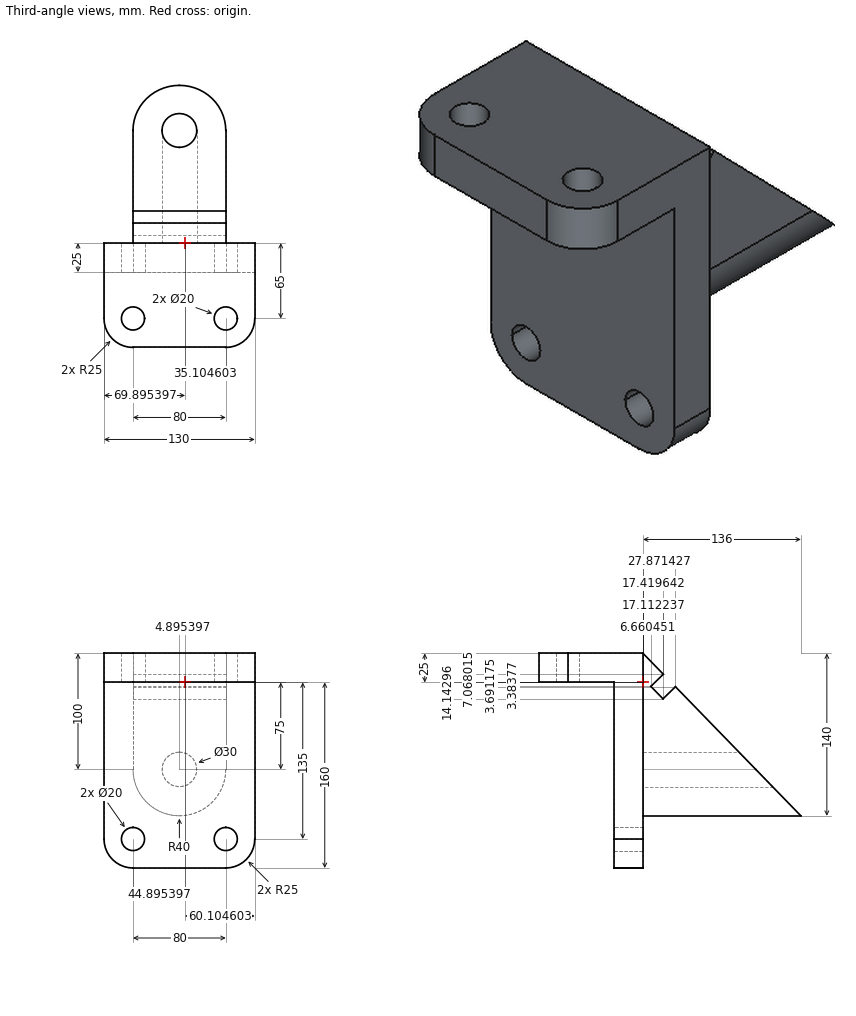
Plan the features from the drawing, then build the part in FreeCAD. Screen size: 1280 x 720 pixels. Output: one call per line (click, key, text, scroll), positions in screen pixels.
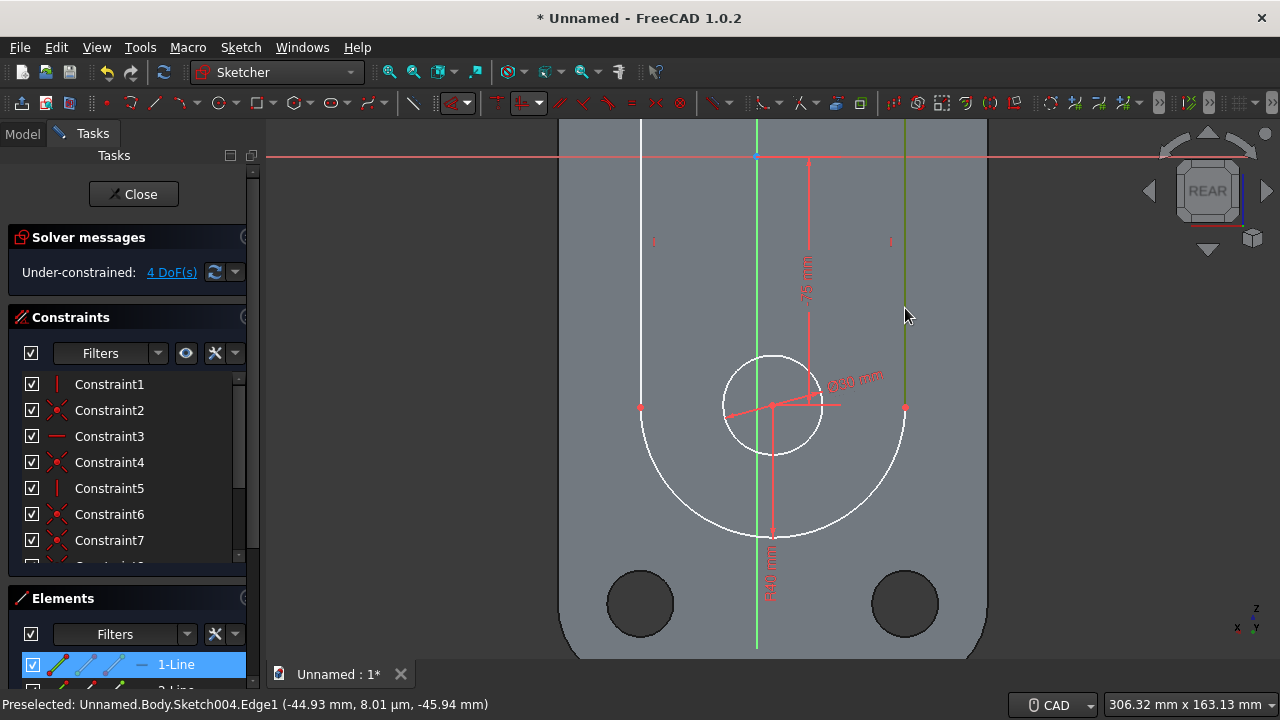
click(470, 104)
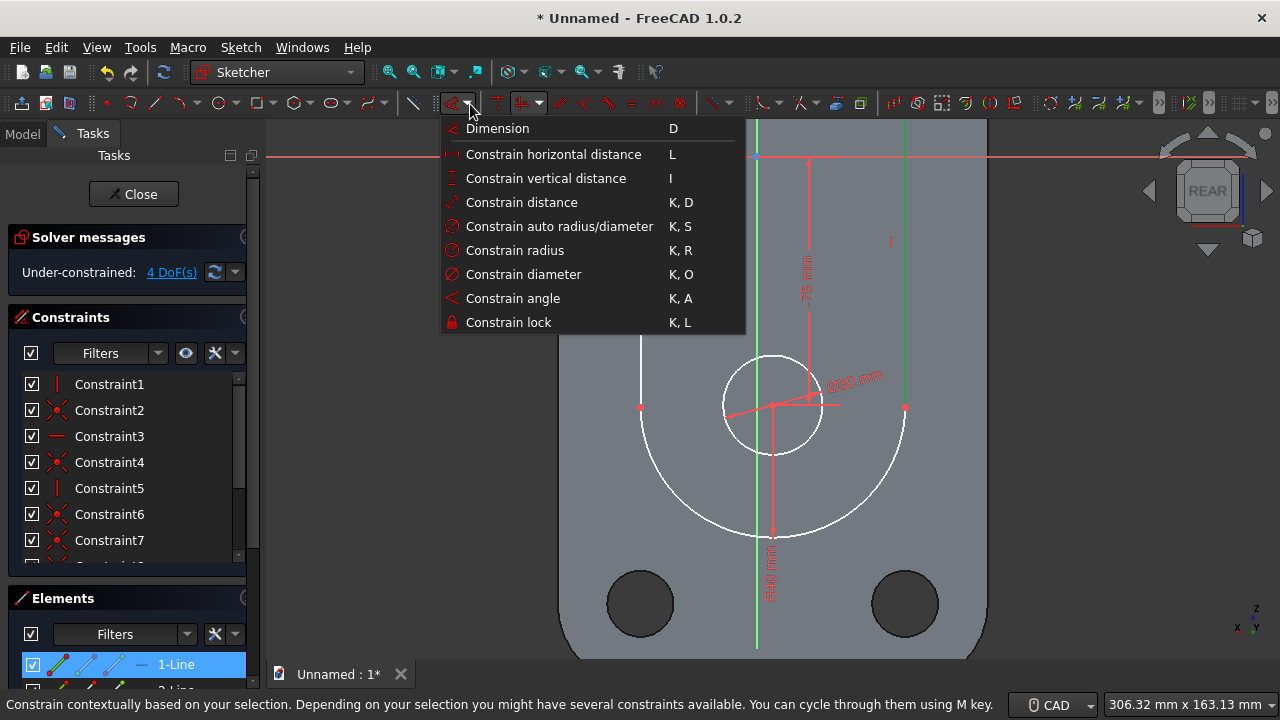
click(593, 178)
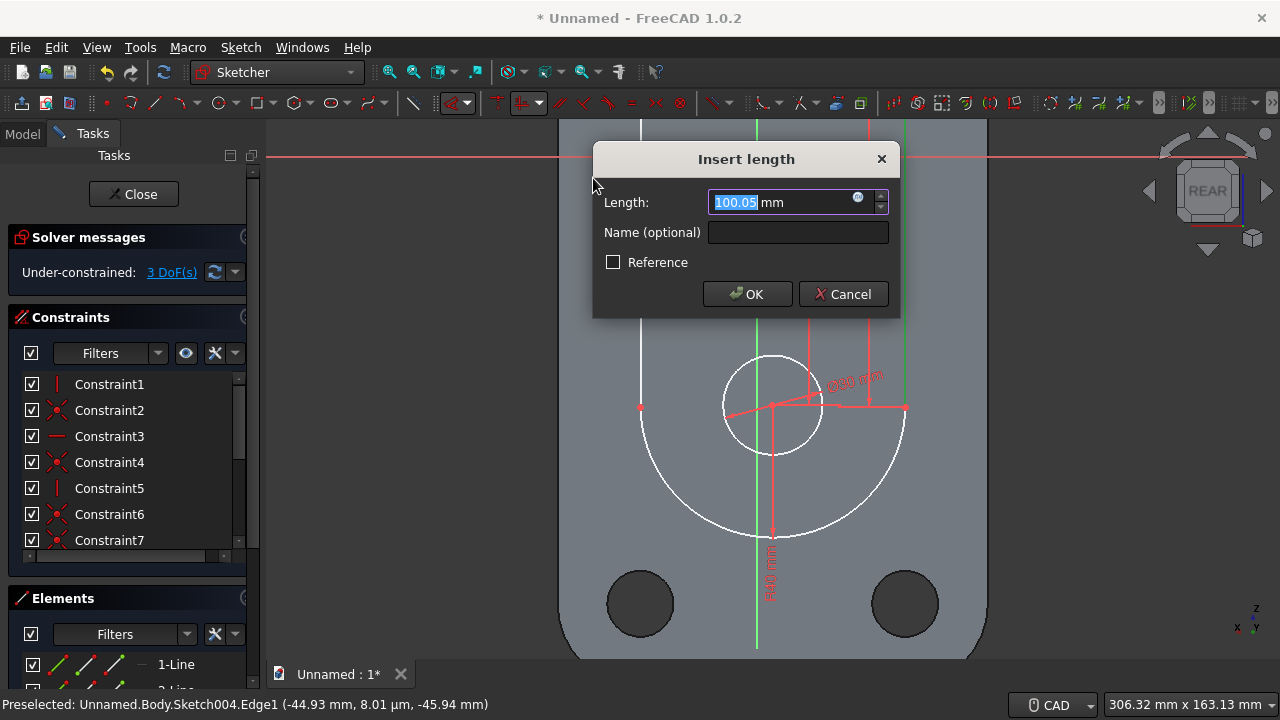
text(100)
key(Return)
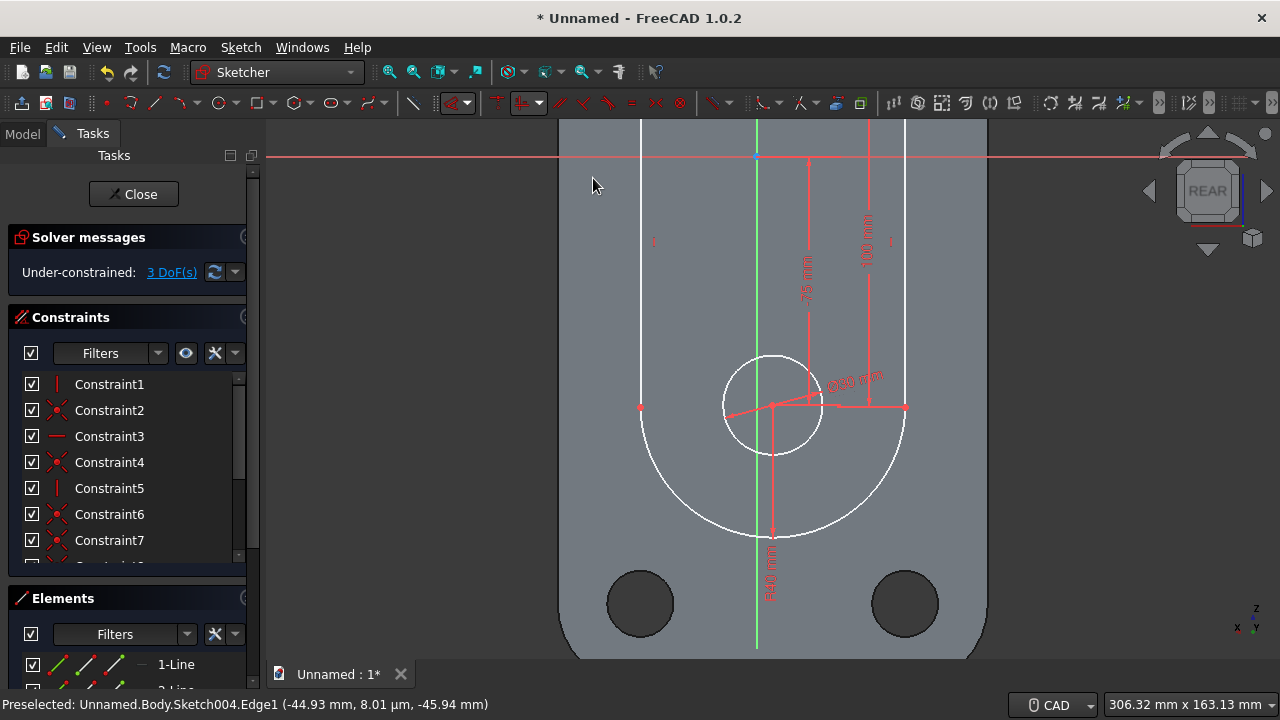
click(641, 175)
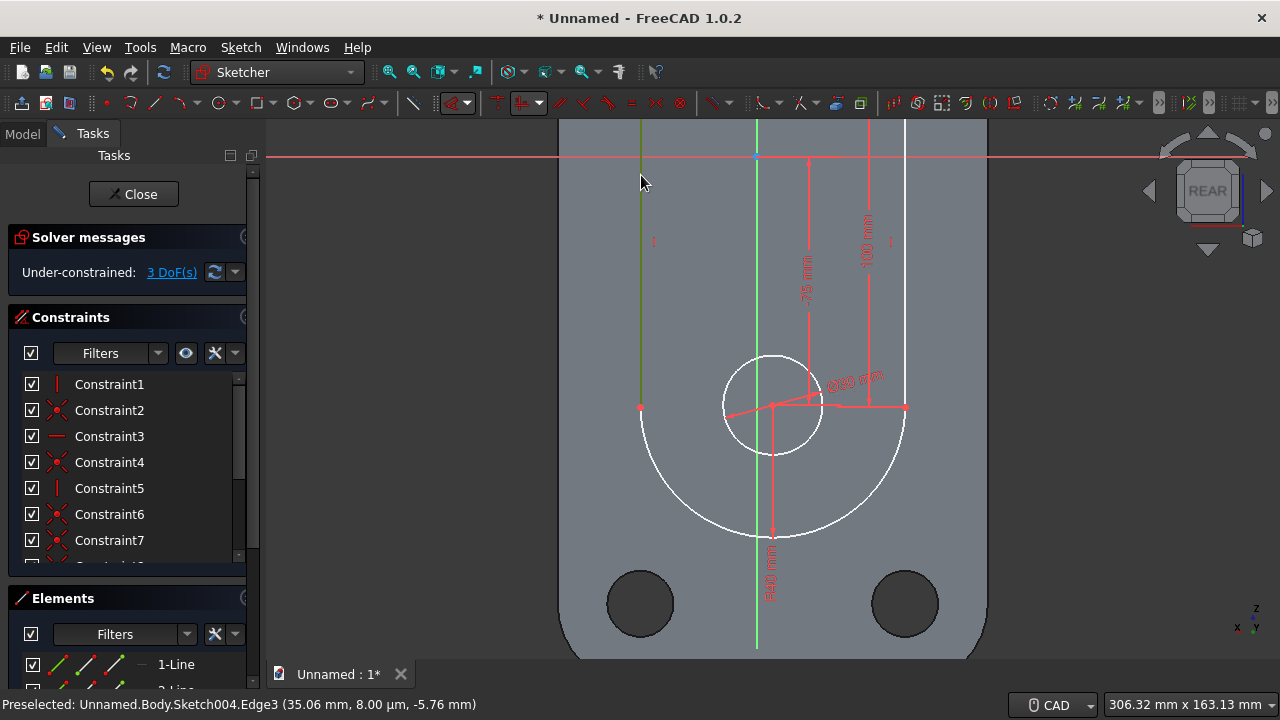
key(i)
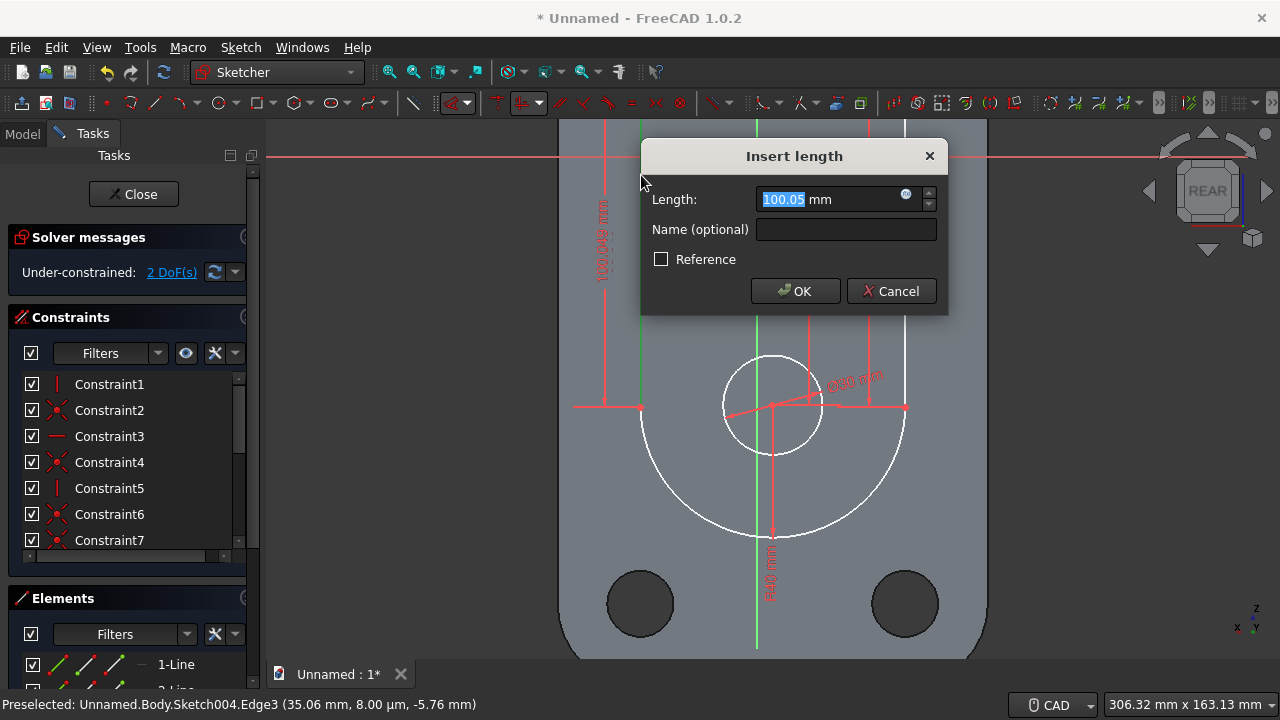
text(100)
key(Return)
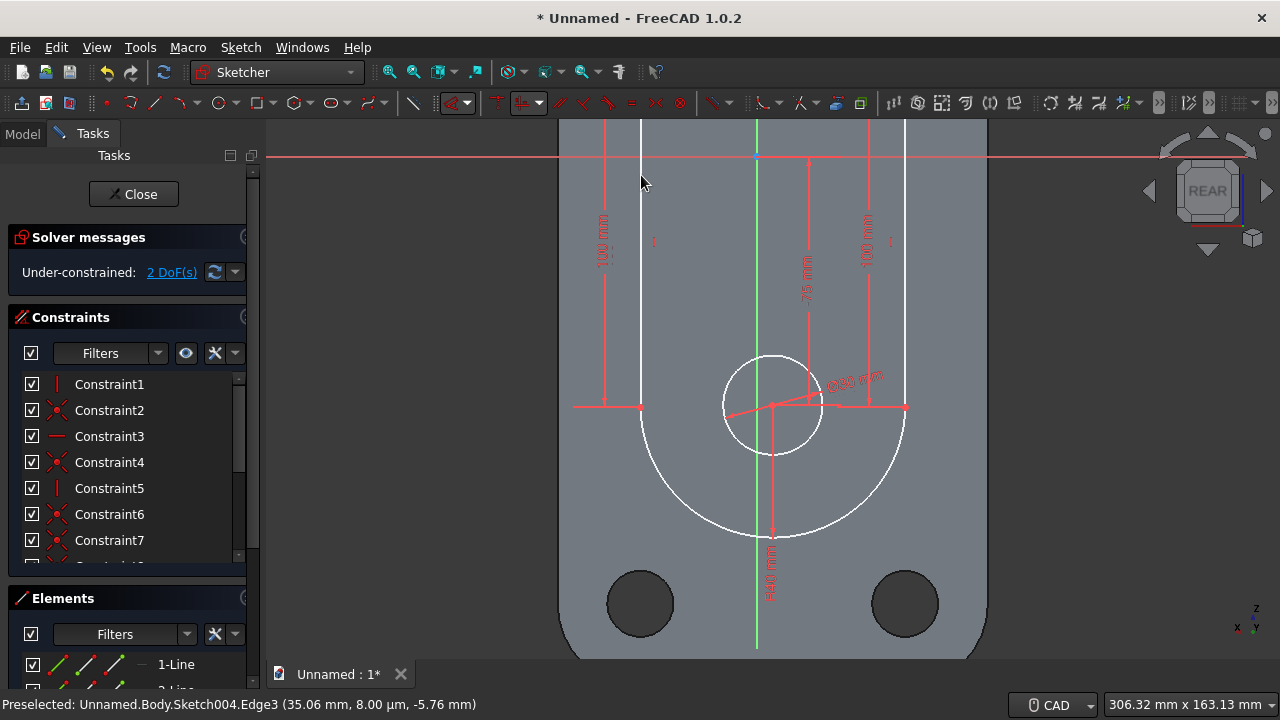
click(905, 407)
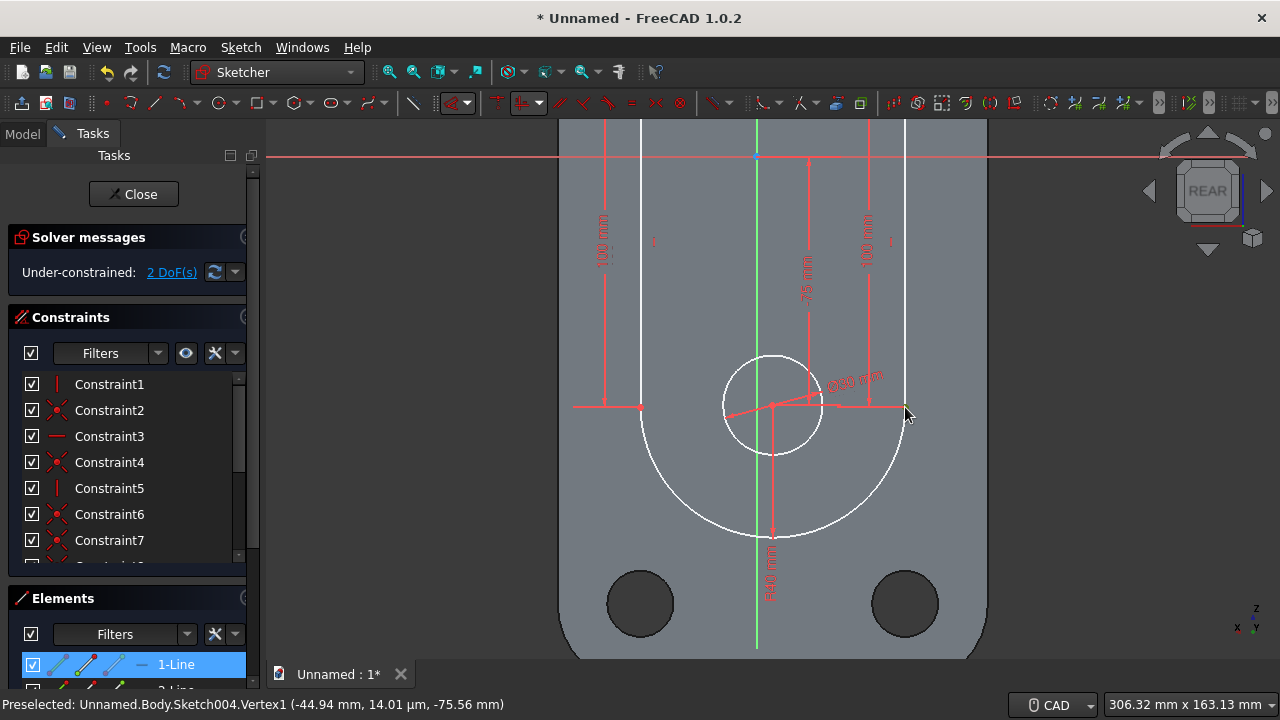
key(i)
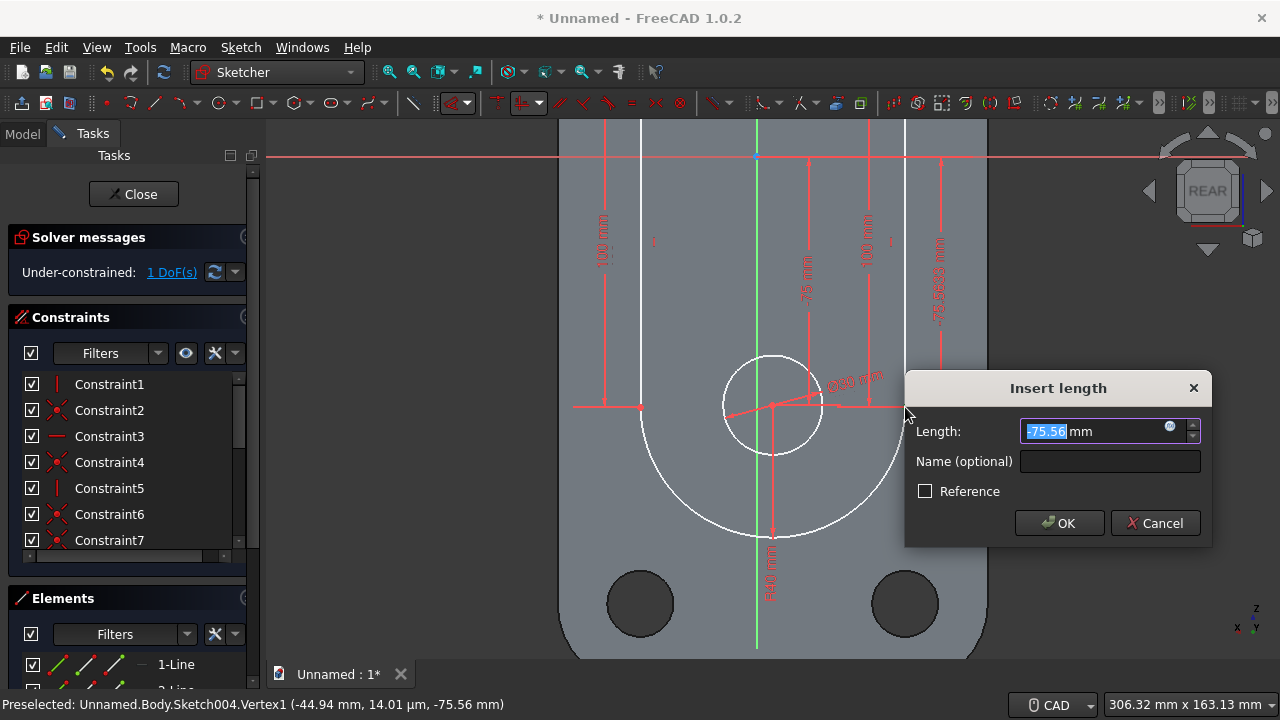
text(-75)
key(Return)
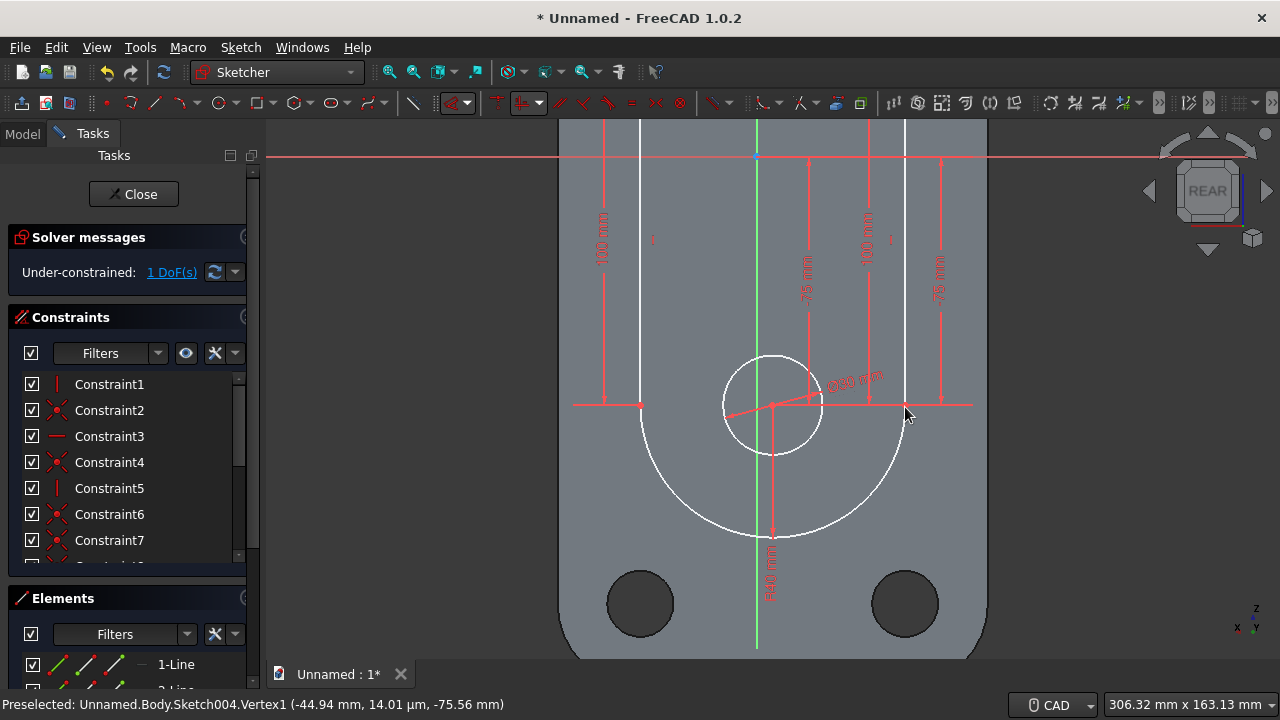
scroll(773, 405, up, 5)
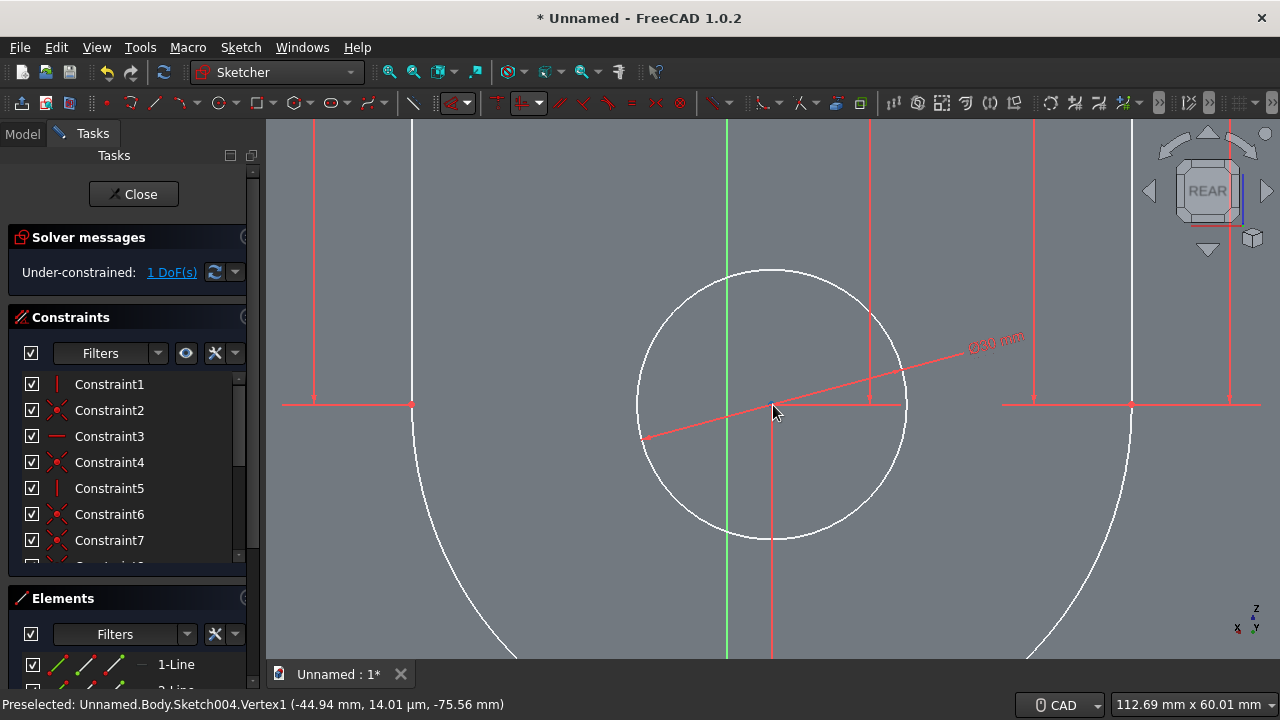
click(772, 405)